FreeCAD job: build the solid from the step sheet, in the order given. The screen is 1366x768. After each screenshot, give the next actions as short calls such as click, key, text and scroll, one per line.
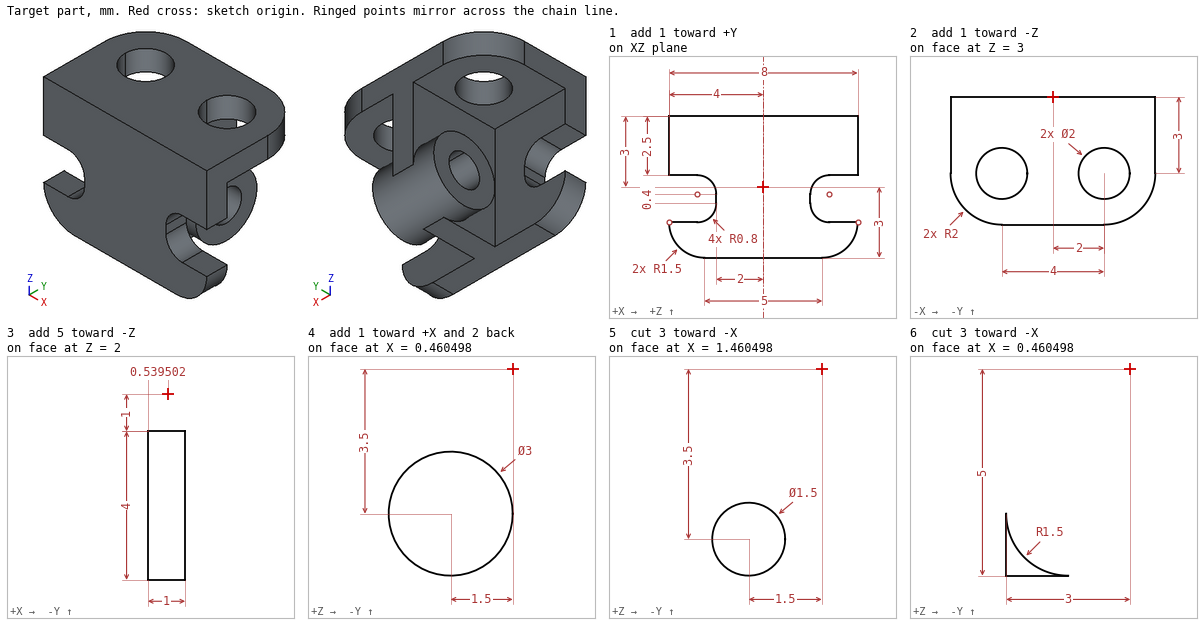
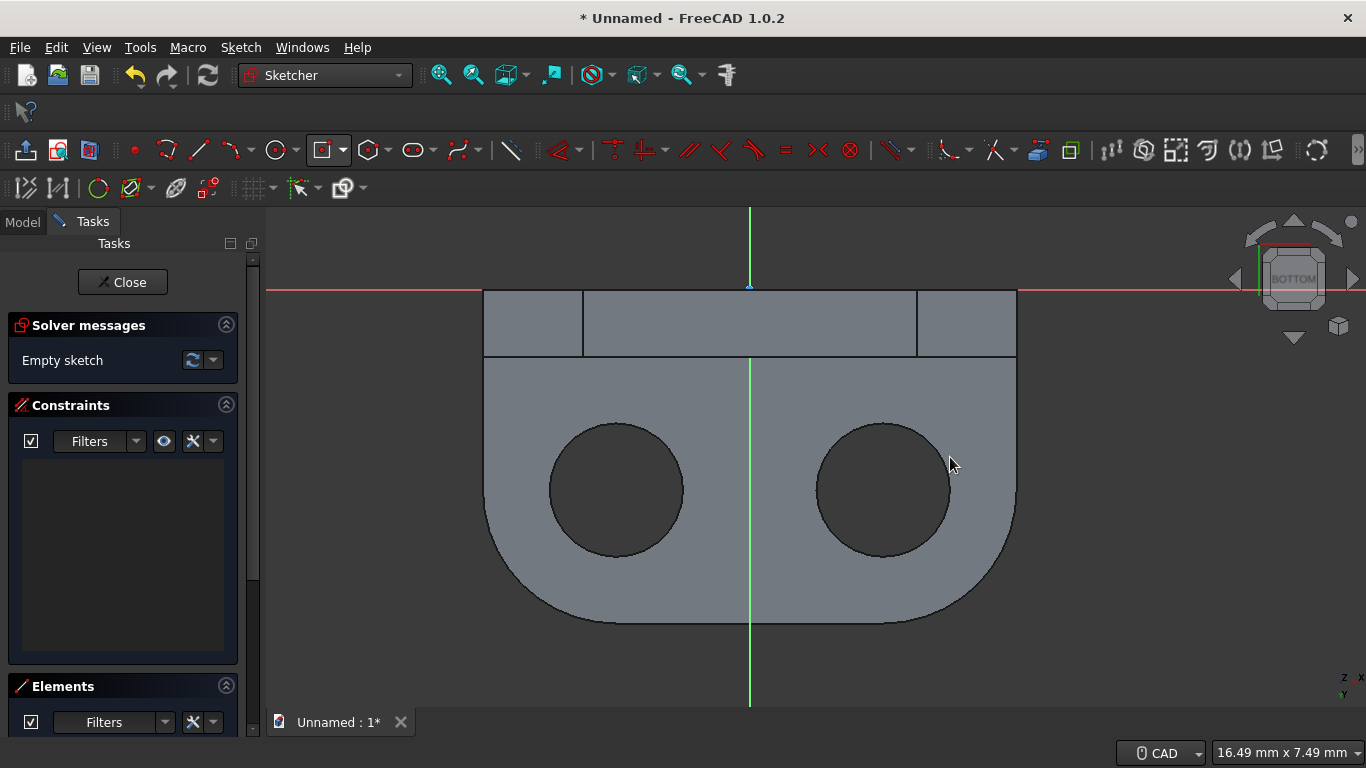
click(346, 150)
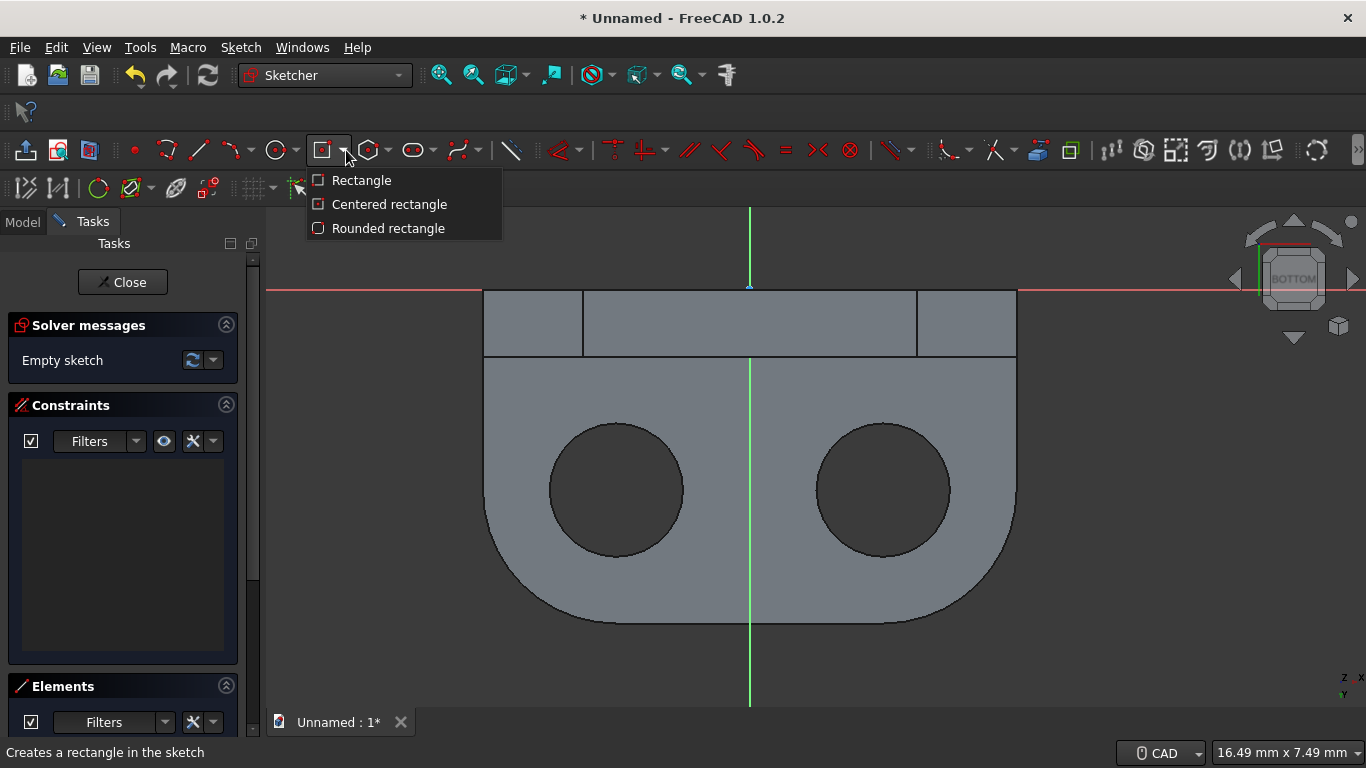
click(404, 180)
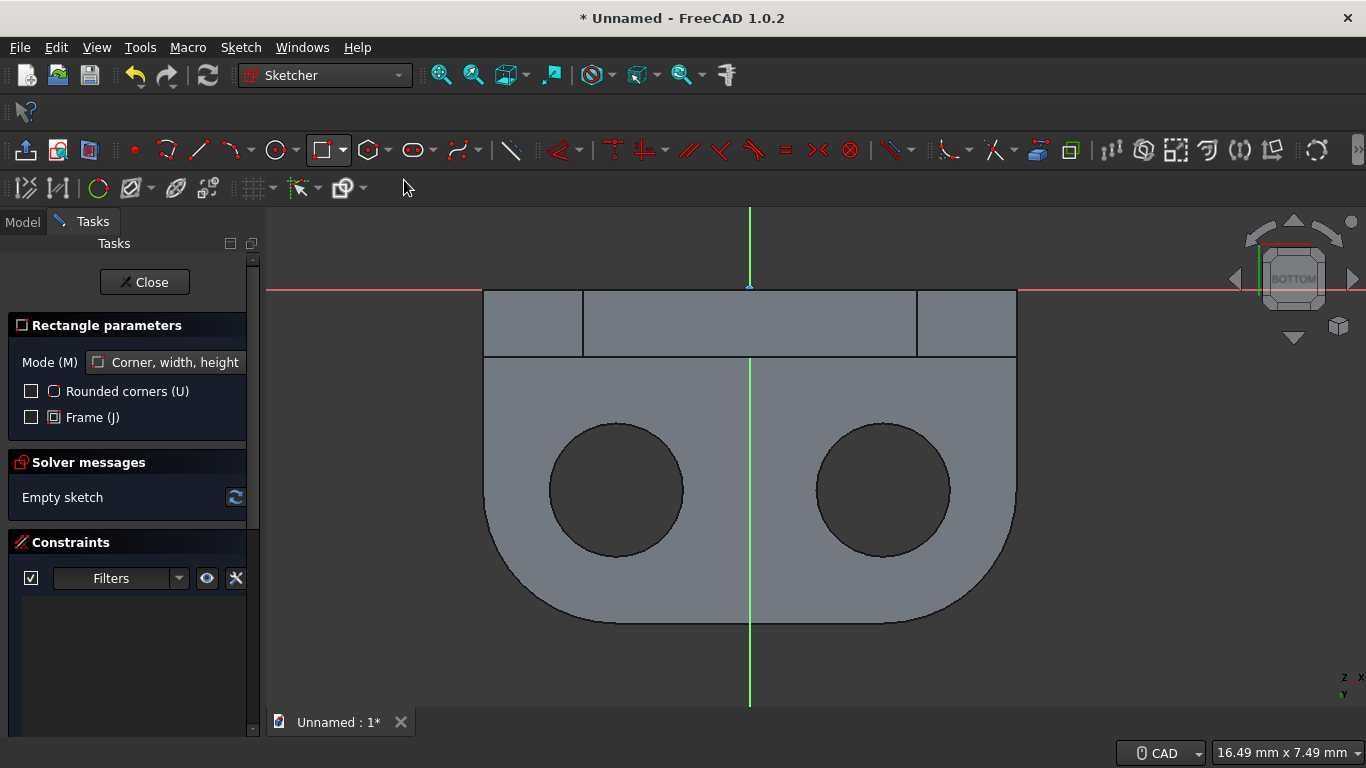
click(714, 357)
click(781, 624)
key(Escape)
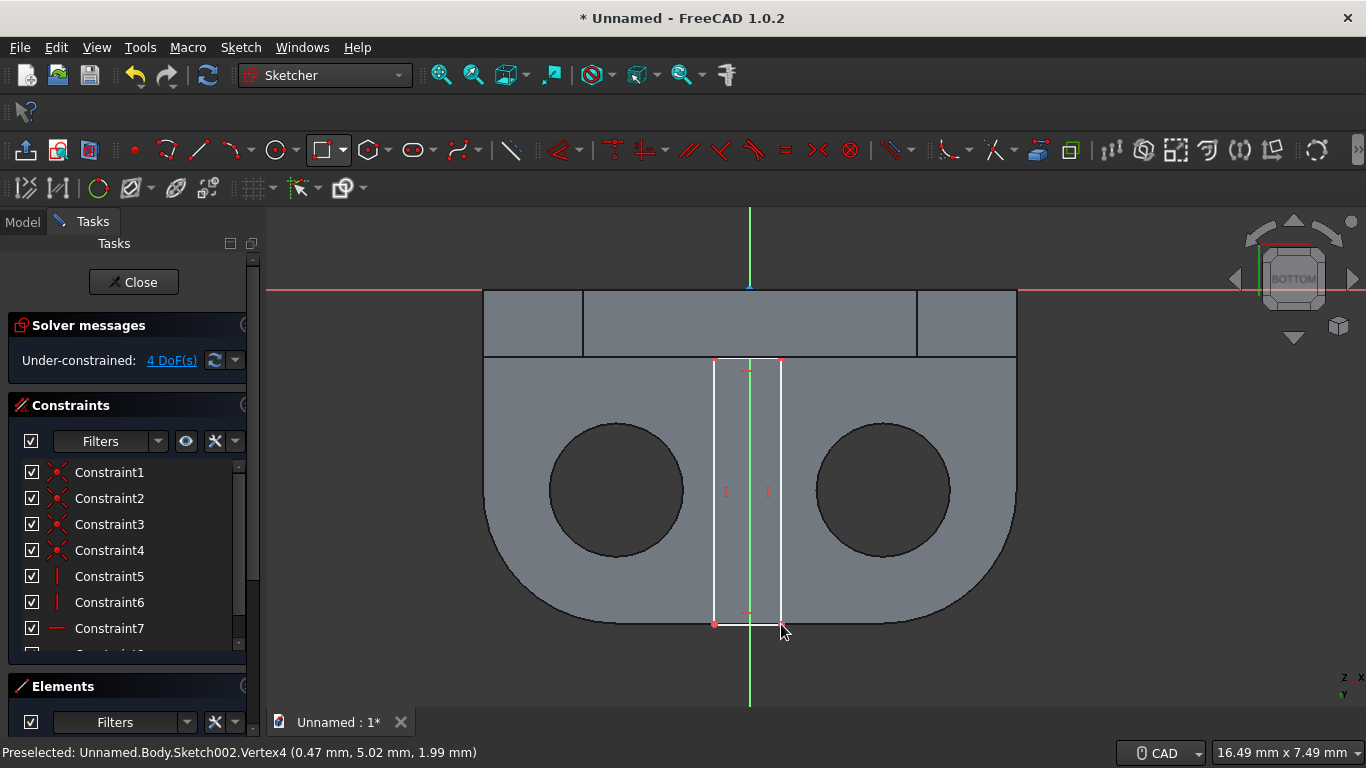
click(558, 150)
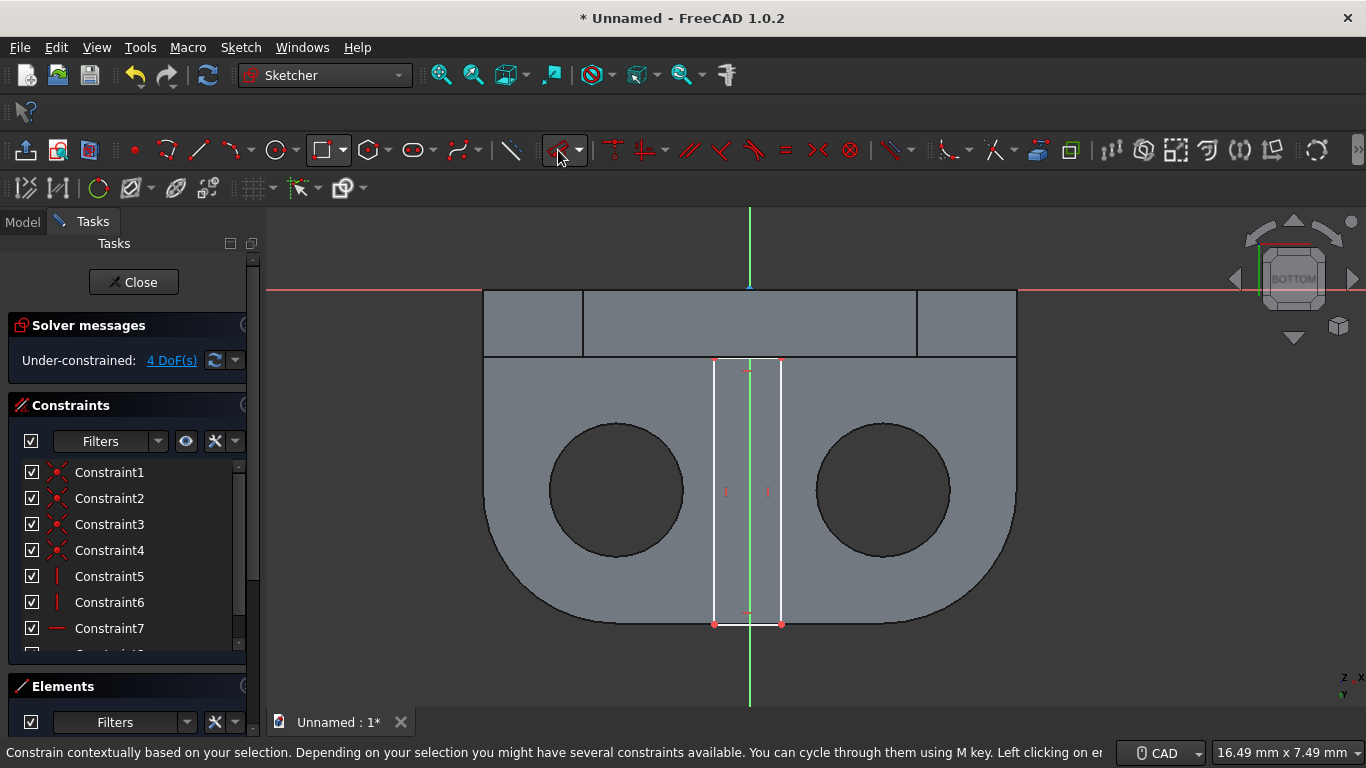
click(714, 438)
click(680, 491)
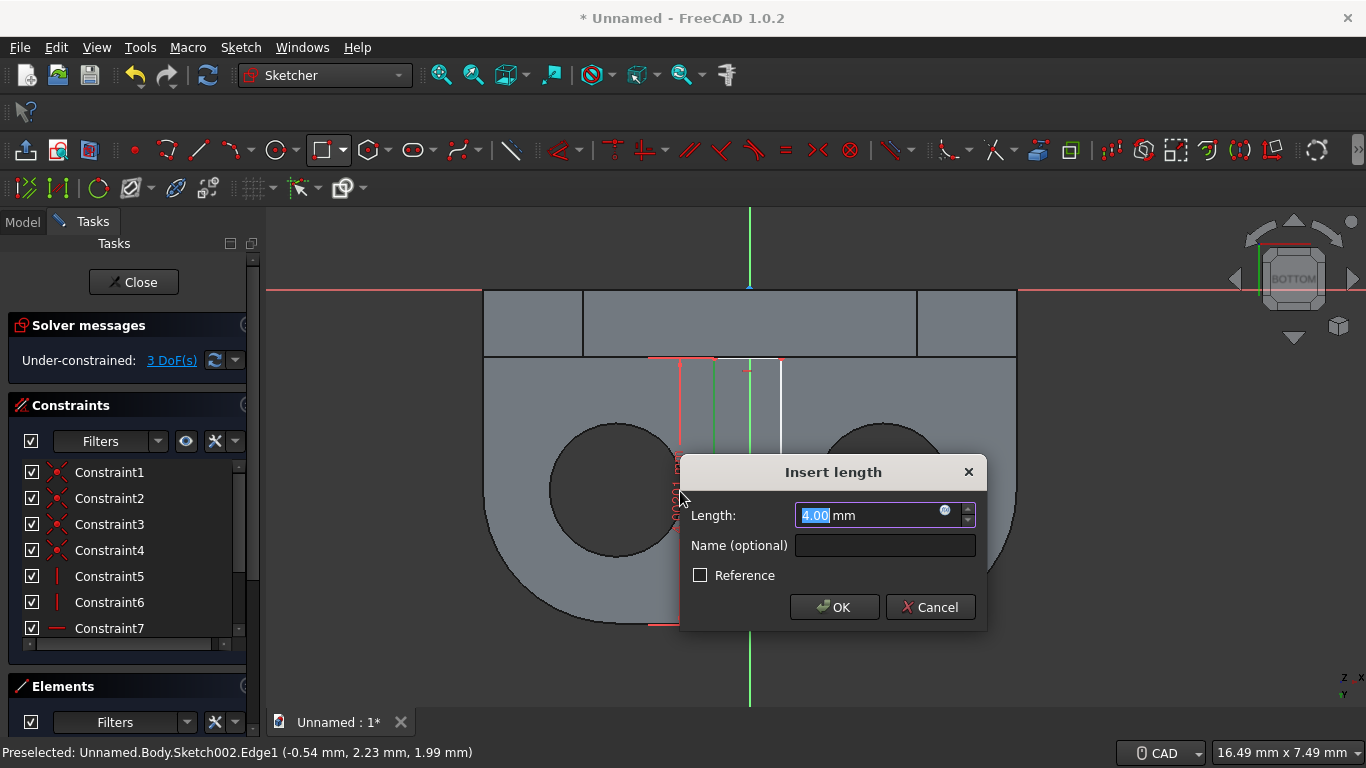
text(4)
key(Return)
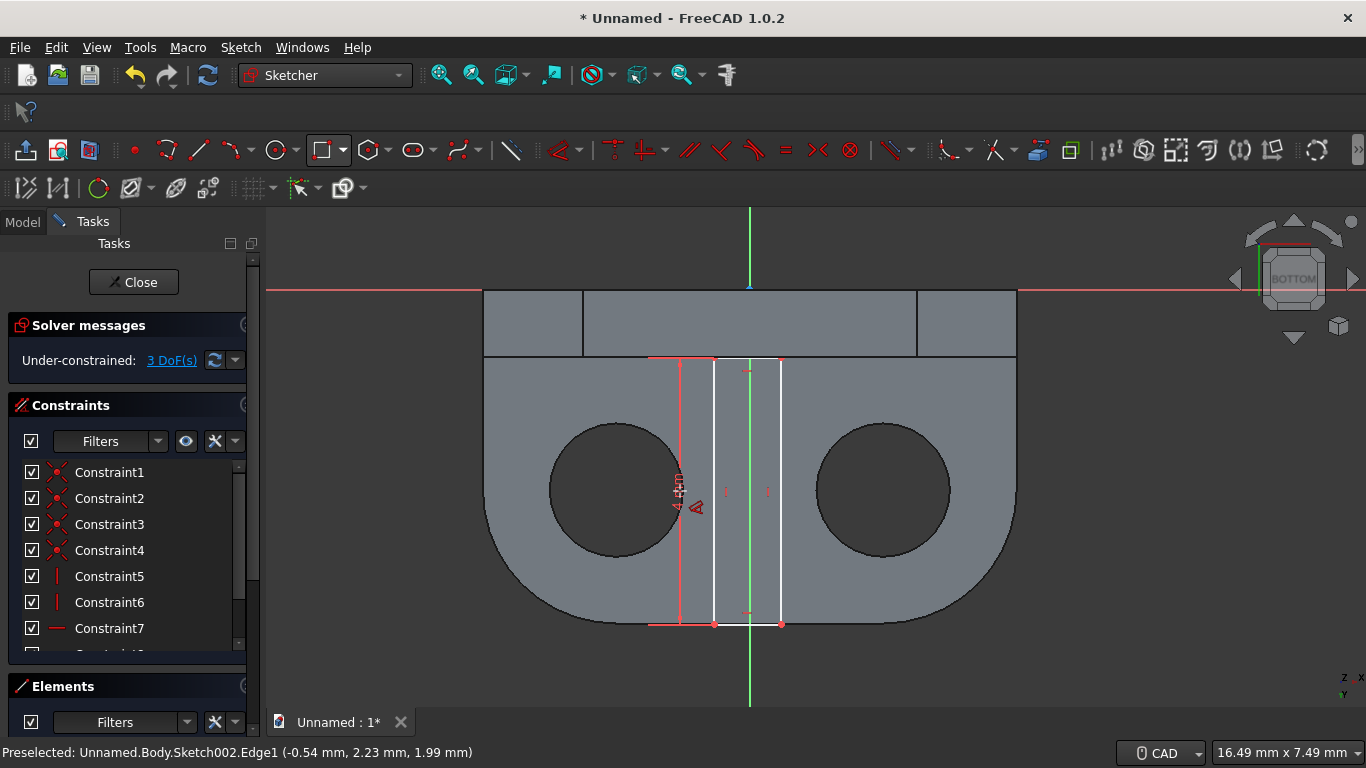
click(734, 625)
click(732, 659)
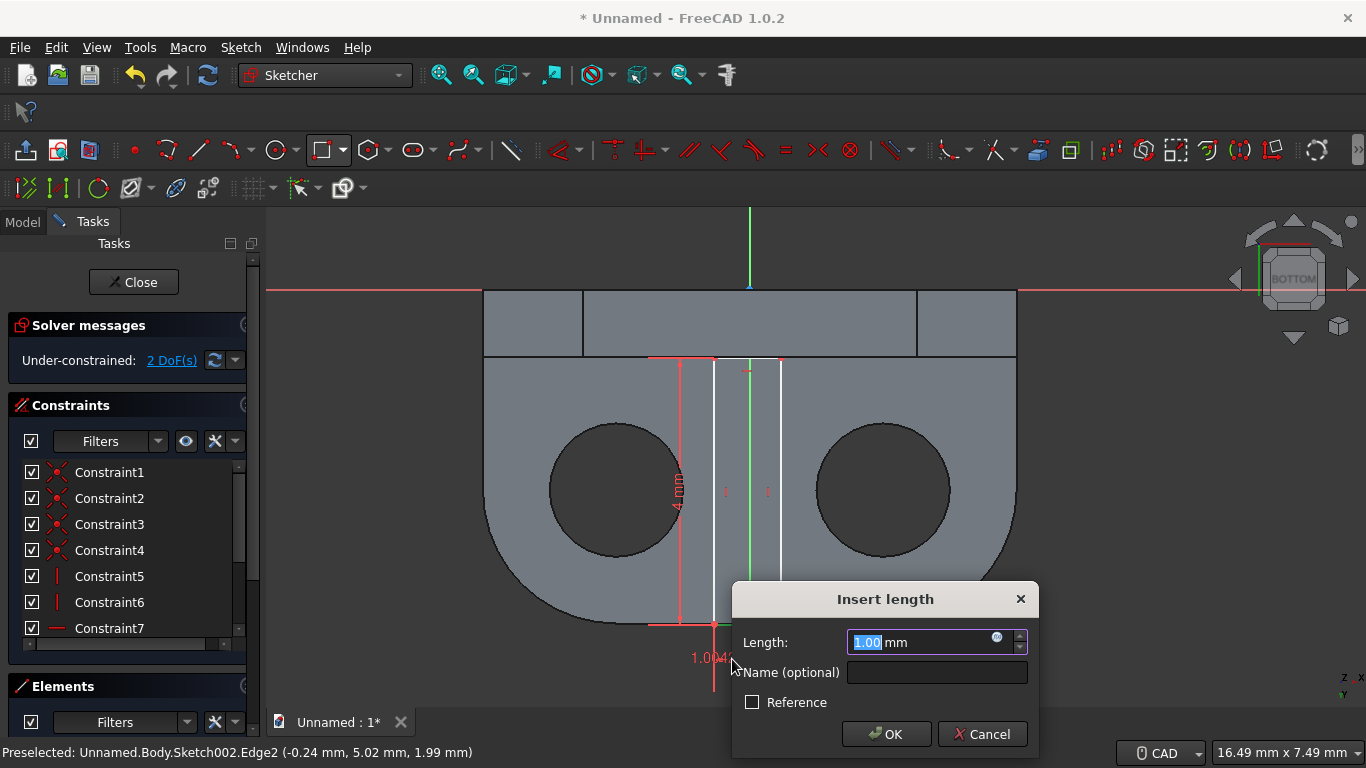
text(1)
key(Return)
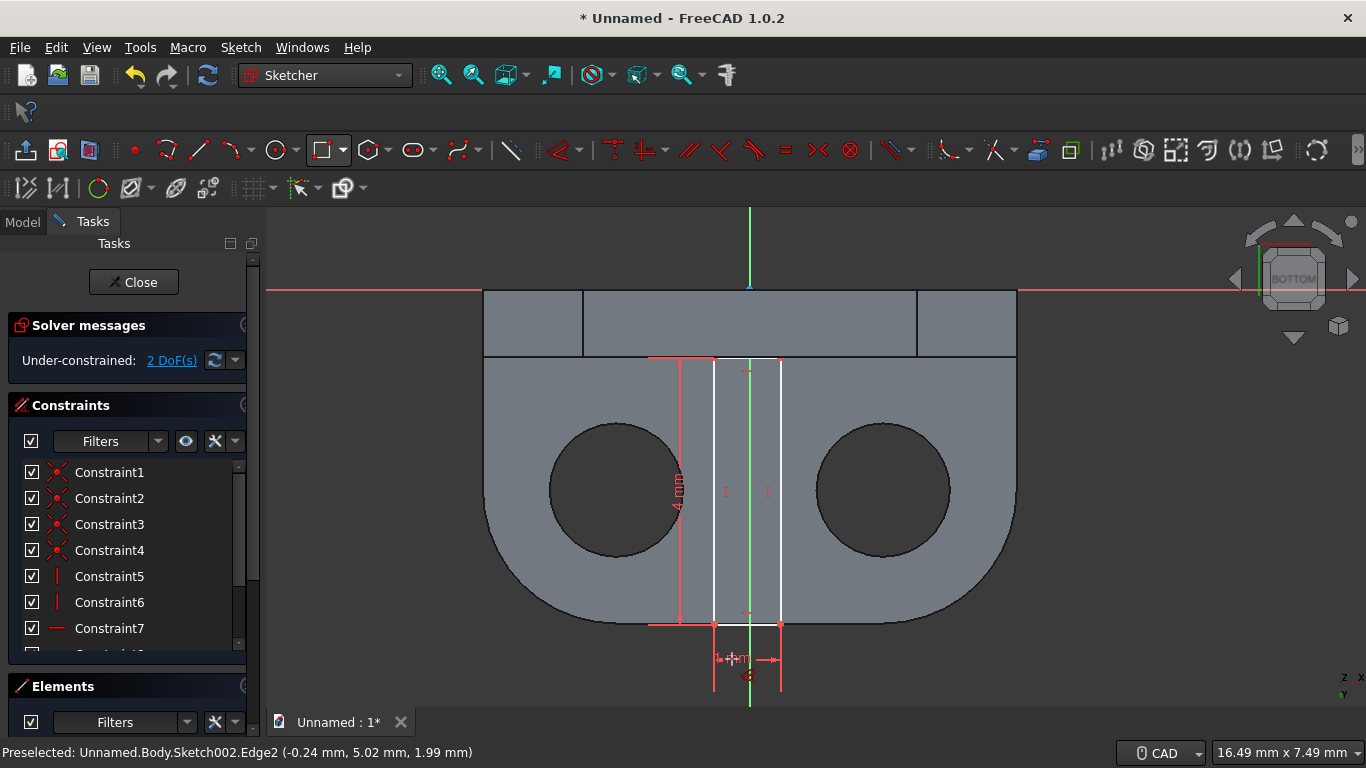
click(714, 358)
click(680, 324)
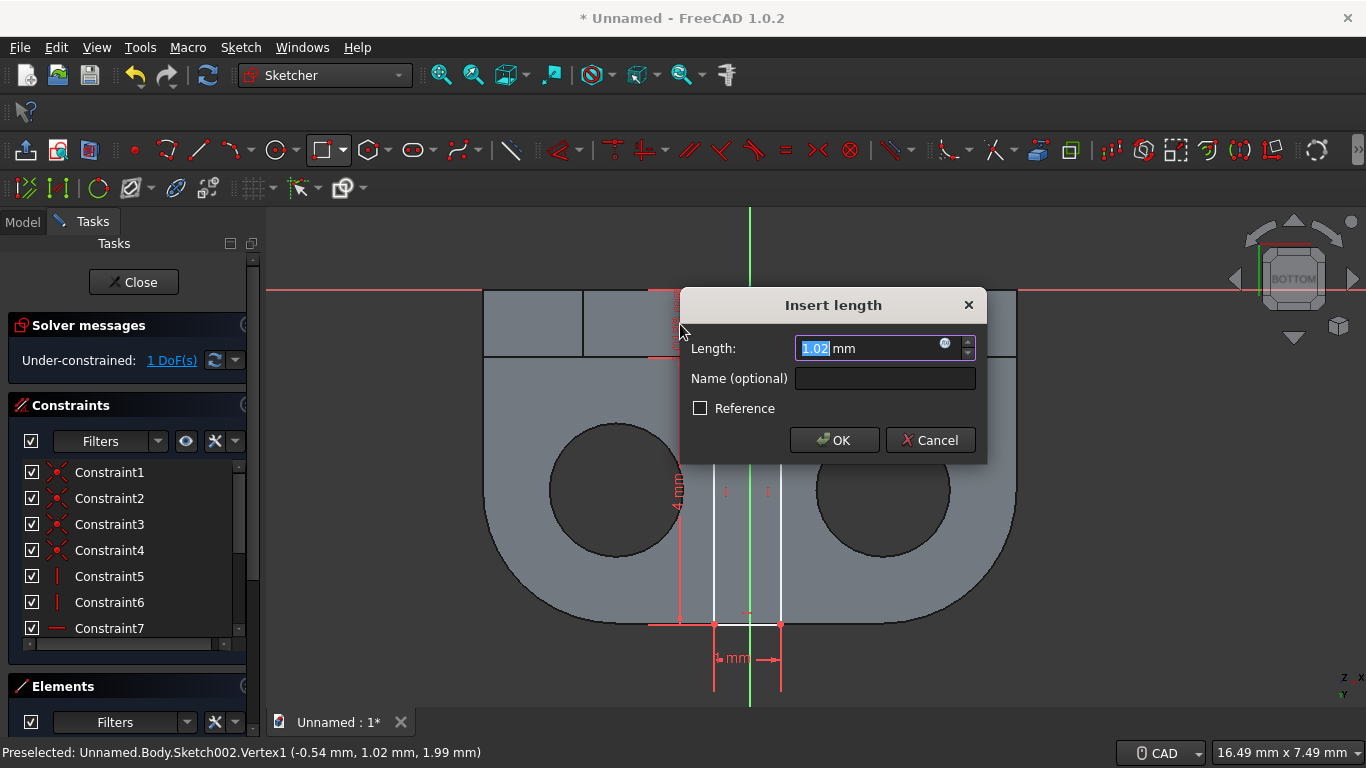
text(1)
key(Return)